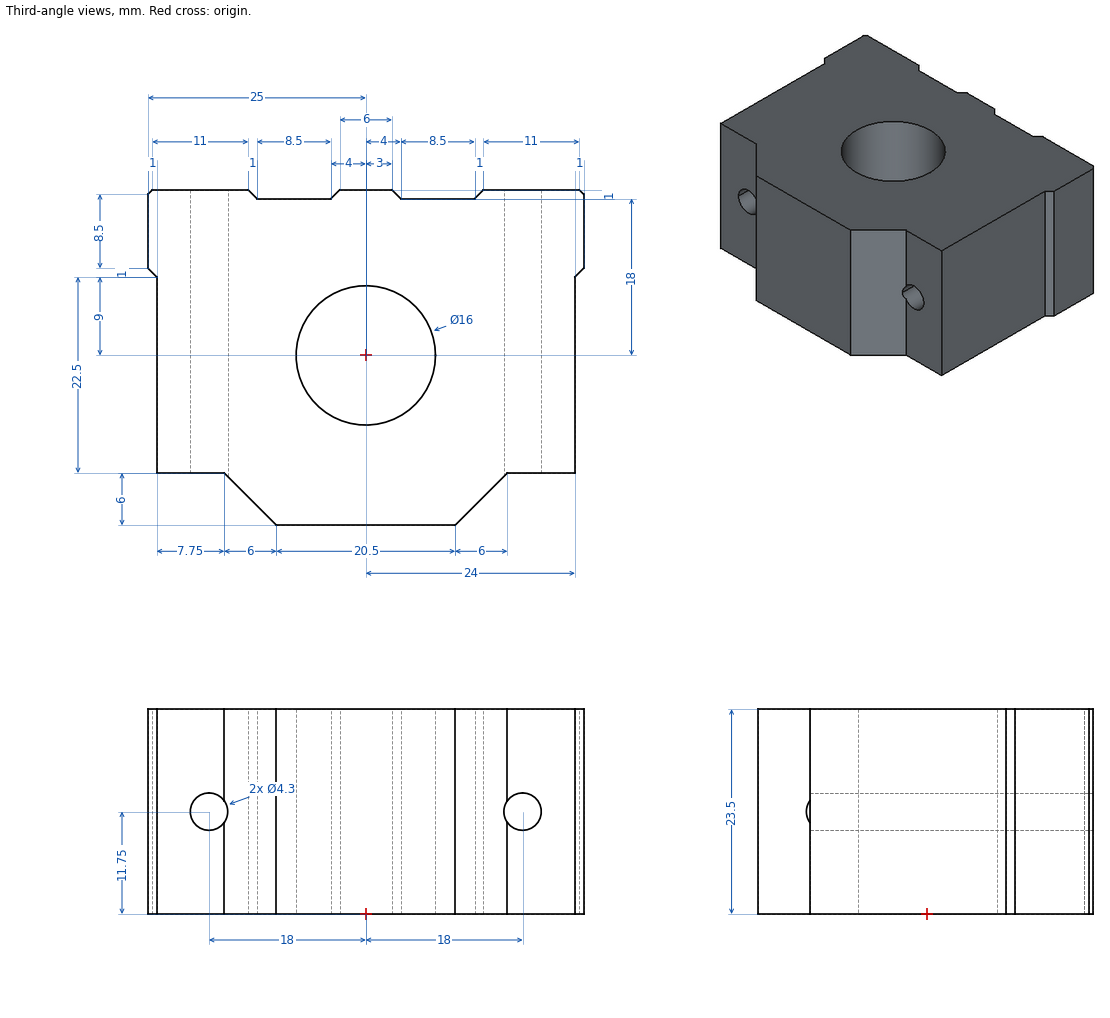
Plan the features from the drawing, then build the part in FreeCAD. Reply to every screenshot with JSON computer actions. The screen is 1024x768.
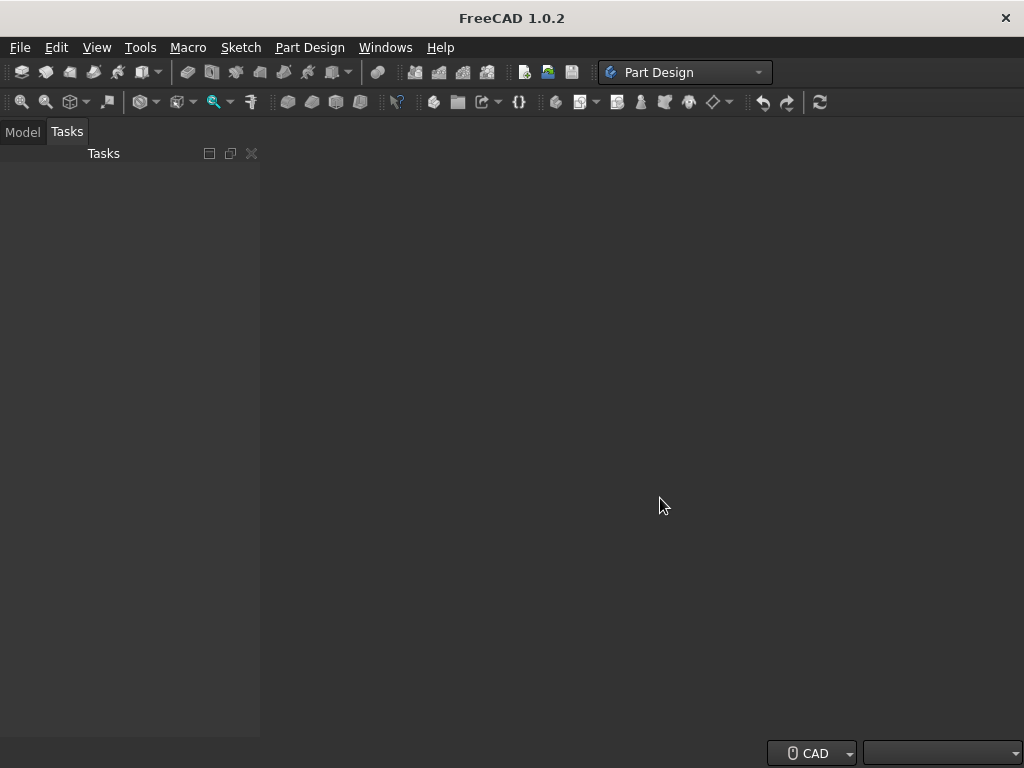
{"action": "left_click", "coordinate": [524, 72]}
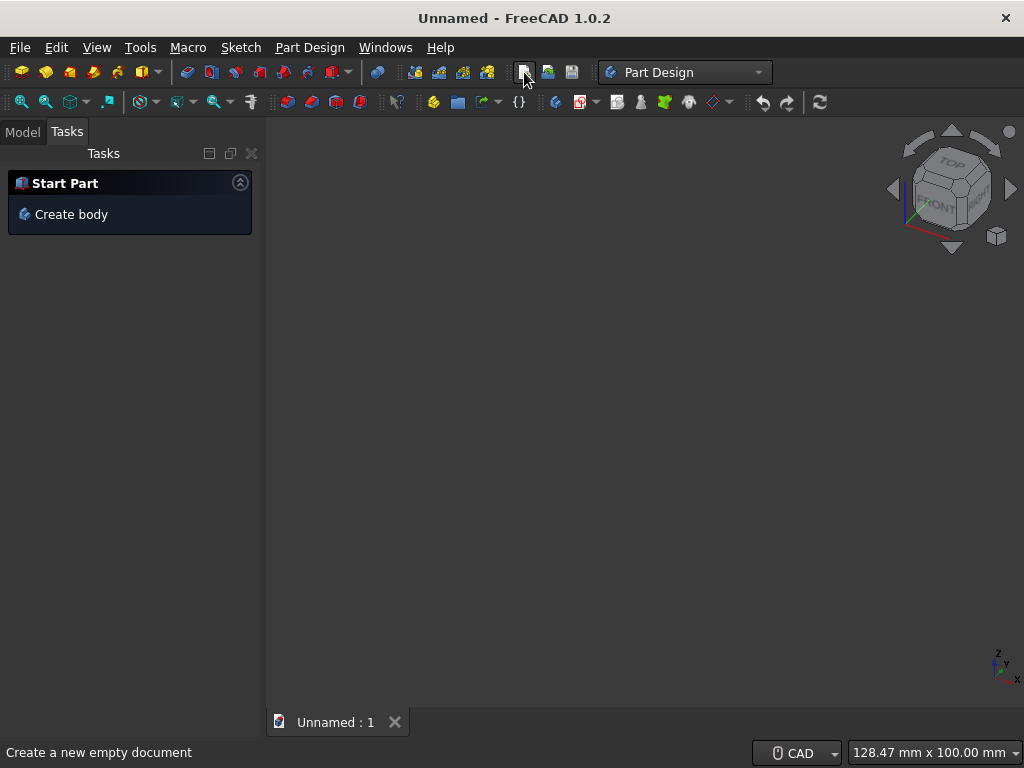
{"action": "left_click", "coordinate": [580, 102]}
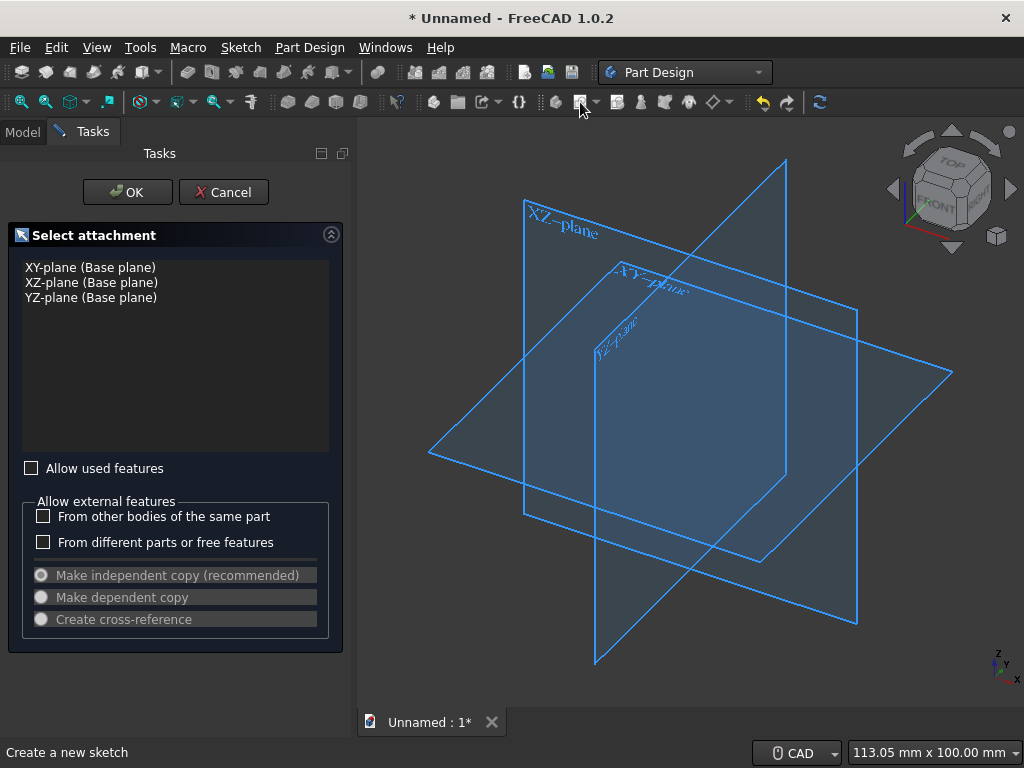
{"action": "left_click", "coordinate": [82, 268]}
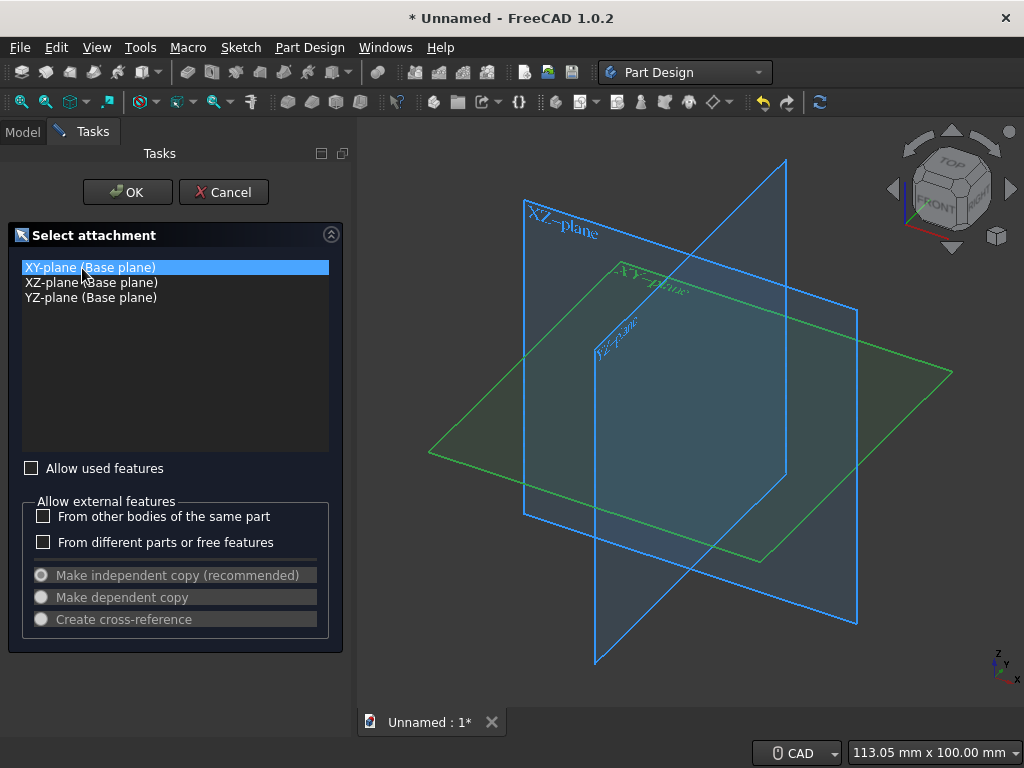
{"action": "left_click", "coordinate": [128, 192]}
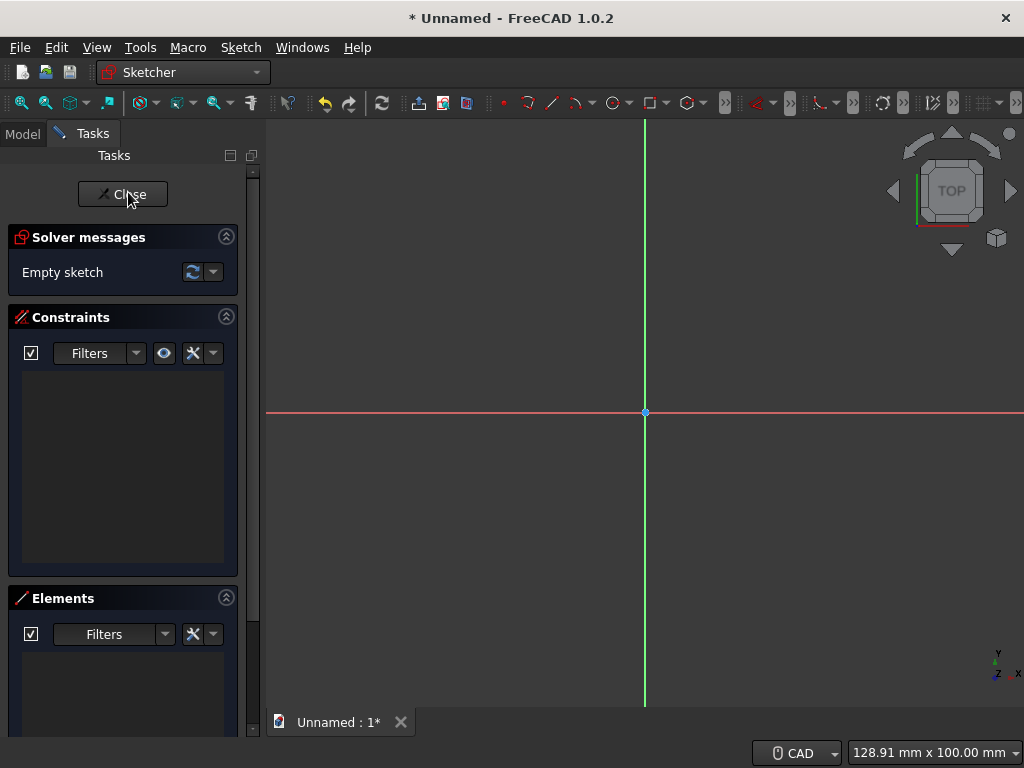
{"action": "scroll", "coordinate": [784, 417], "scroll_direction": "up", "scroll_amount": 2}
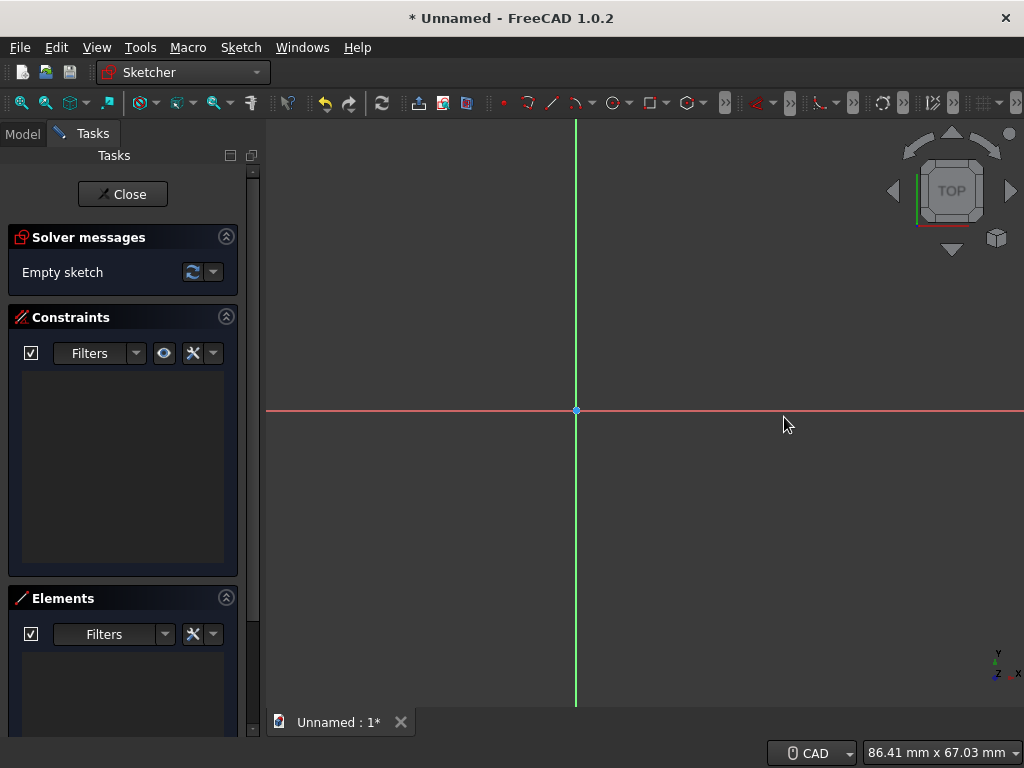
{"action": "left_click", "coordinate": [528, 104]}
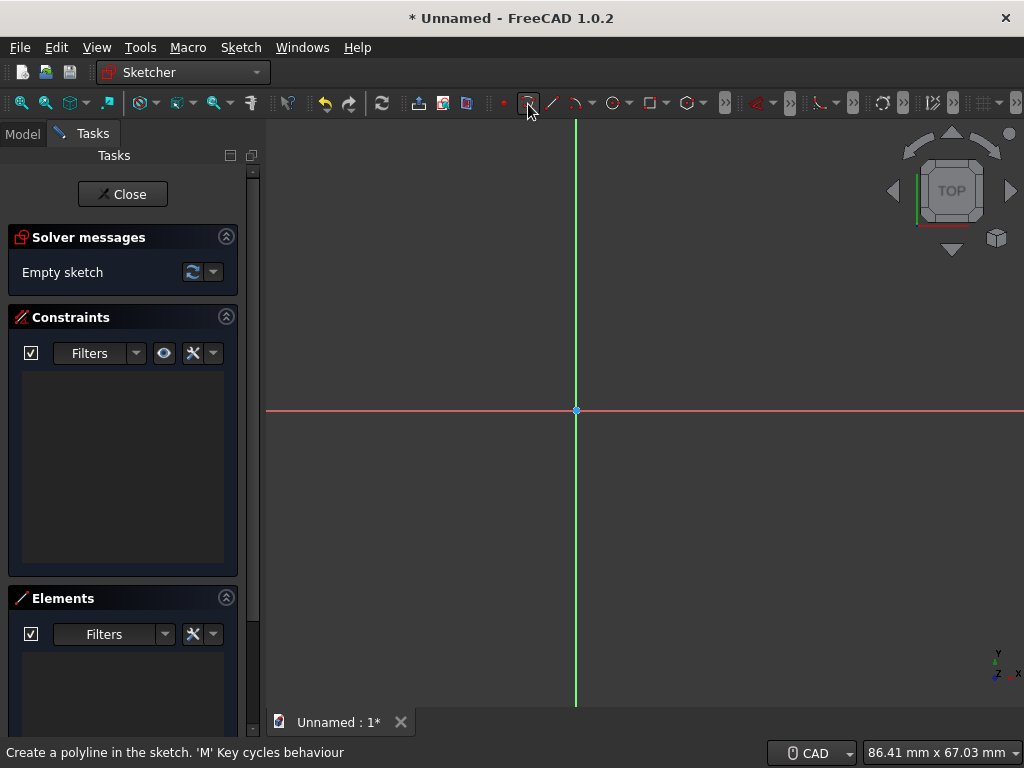
{"action": "left_click", "coordinate": [611, 253]}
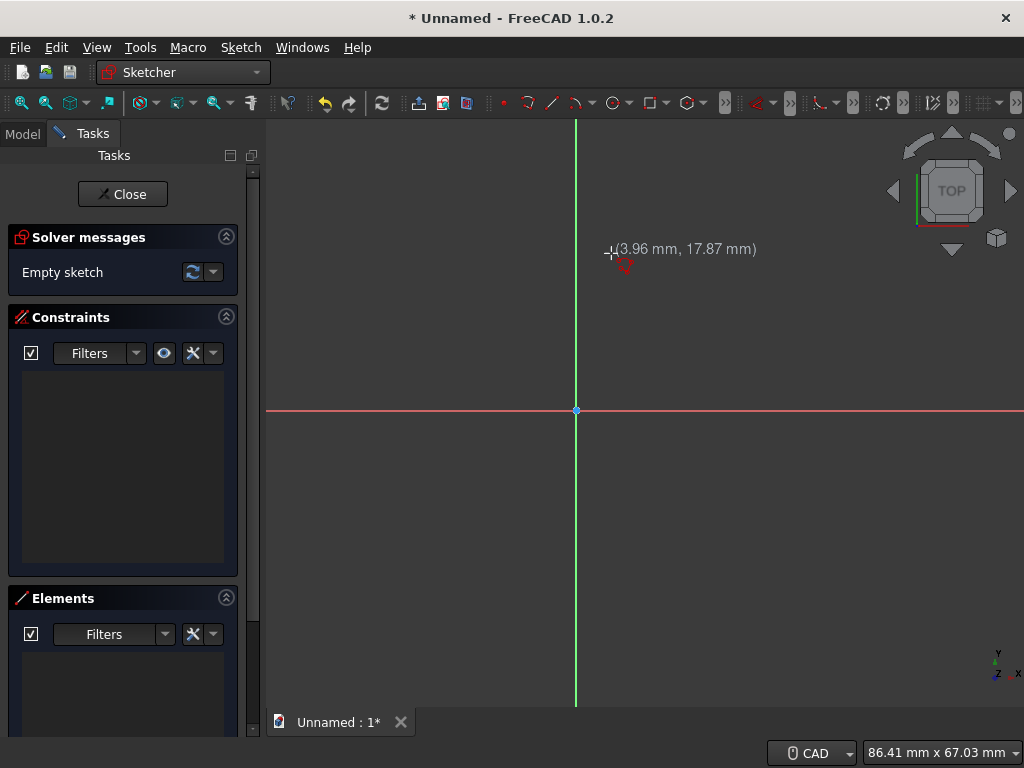
{"action": "scroll", "coordinate": [603, 244], "scroll_direction": "up", "scroll_amount": 2}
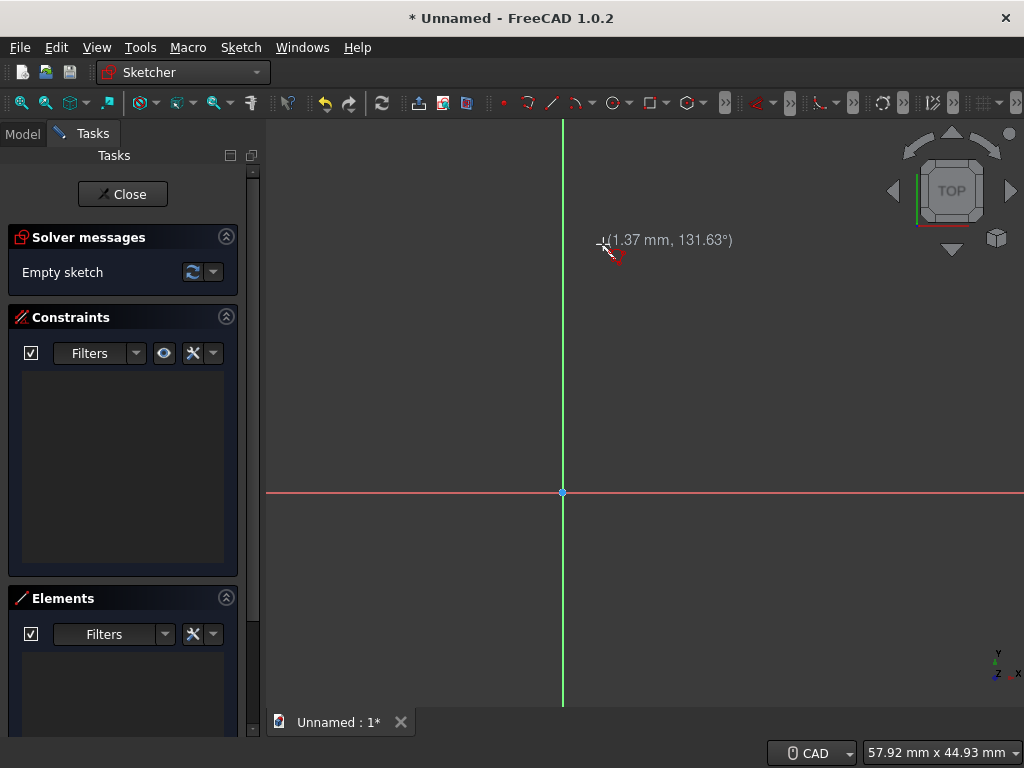
{"action": "left_click", "coordinate": [602, 244]}
{"action": "left_click", "coordinate": [524, 244]}
{"action": "left_click", "coordinate": [511, 257]}
{"action": "left_click", "coordinate": [399, 257]}
{"action": "left_click", "coordinate": [386, 244]}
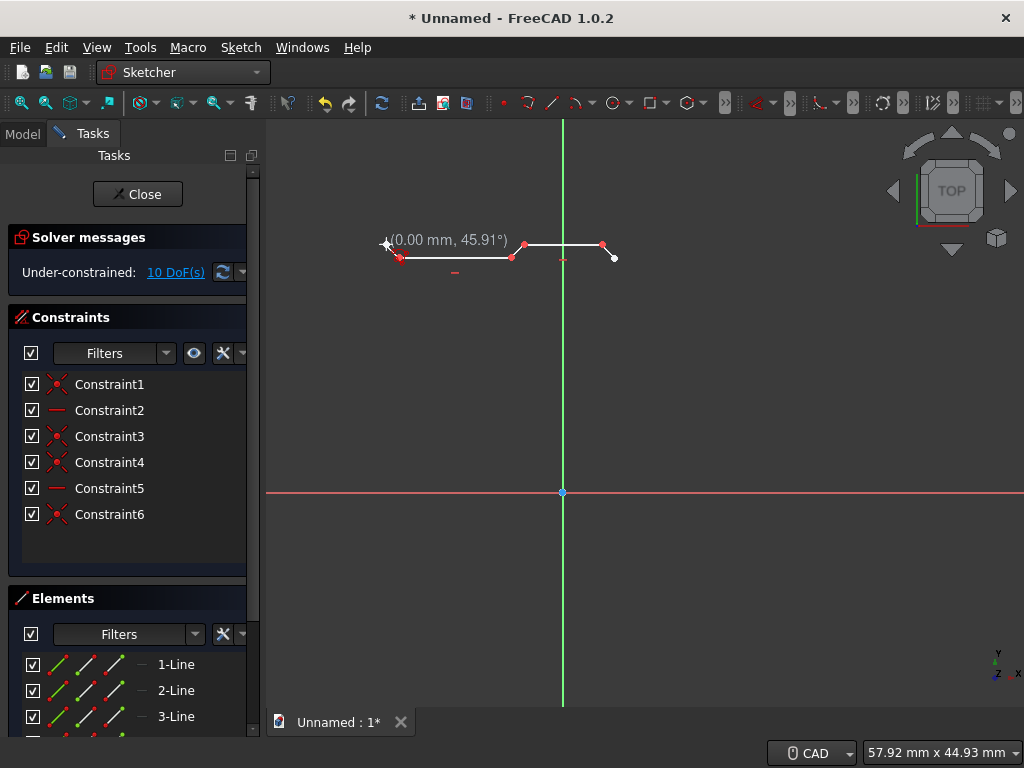
{"action": "scroll", "coordinate": [604, 244], "scroll_direction": "down", "scroll_amount": 2}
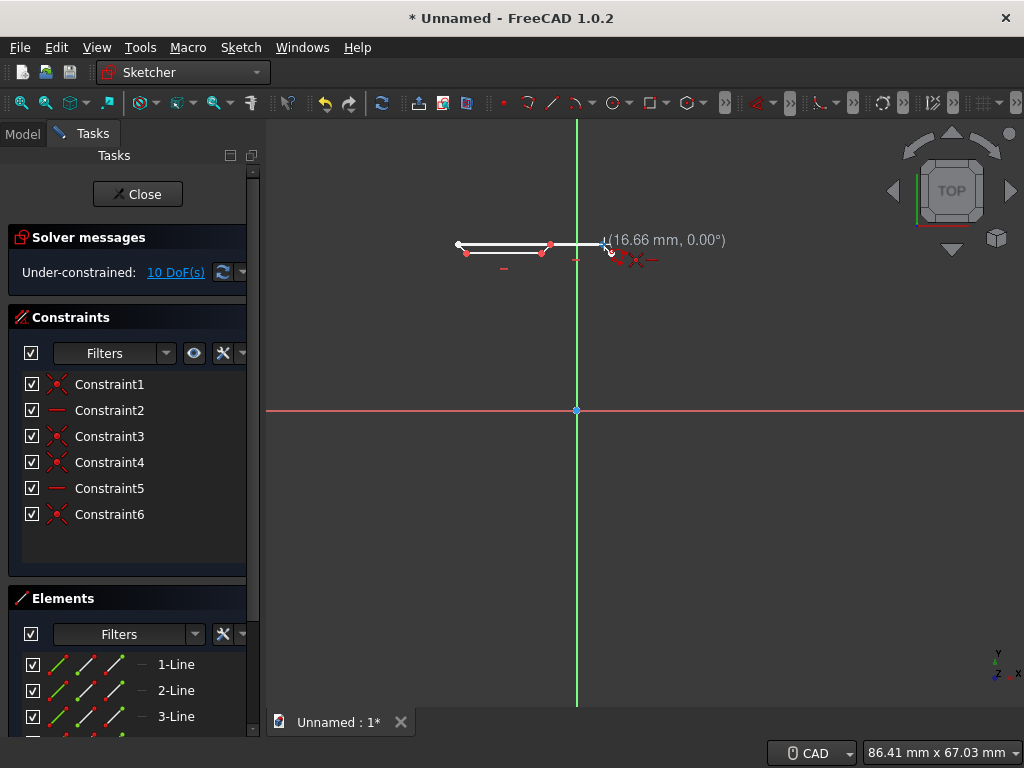
{"action": "left_click", "coordinate": [362, 244]}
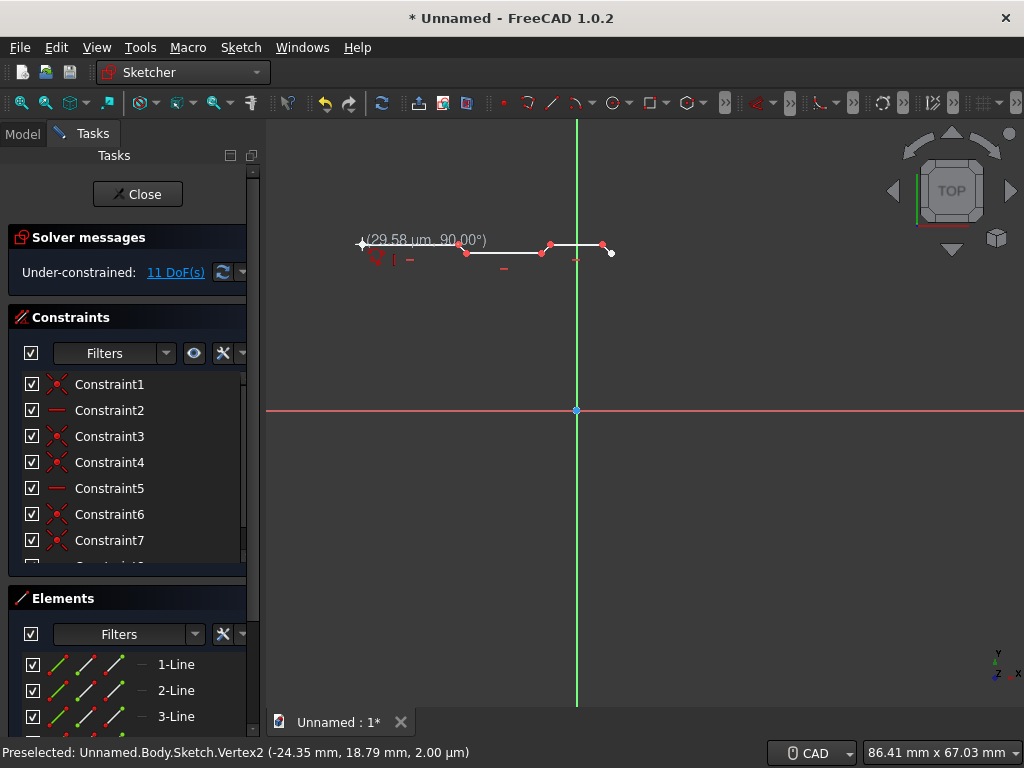
{"action": "scroll", "coordinate": [357, 249], "scroll_direction": "up", "scroll_amount": 5}